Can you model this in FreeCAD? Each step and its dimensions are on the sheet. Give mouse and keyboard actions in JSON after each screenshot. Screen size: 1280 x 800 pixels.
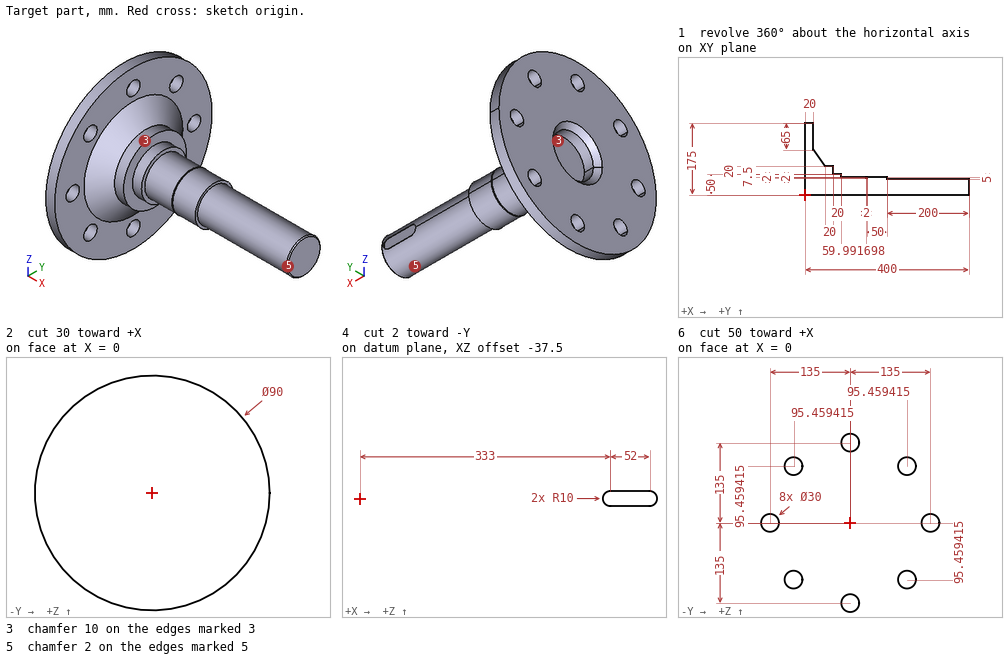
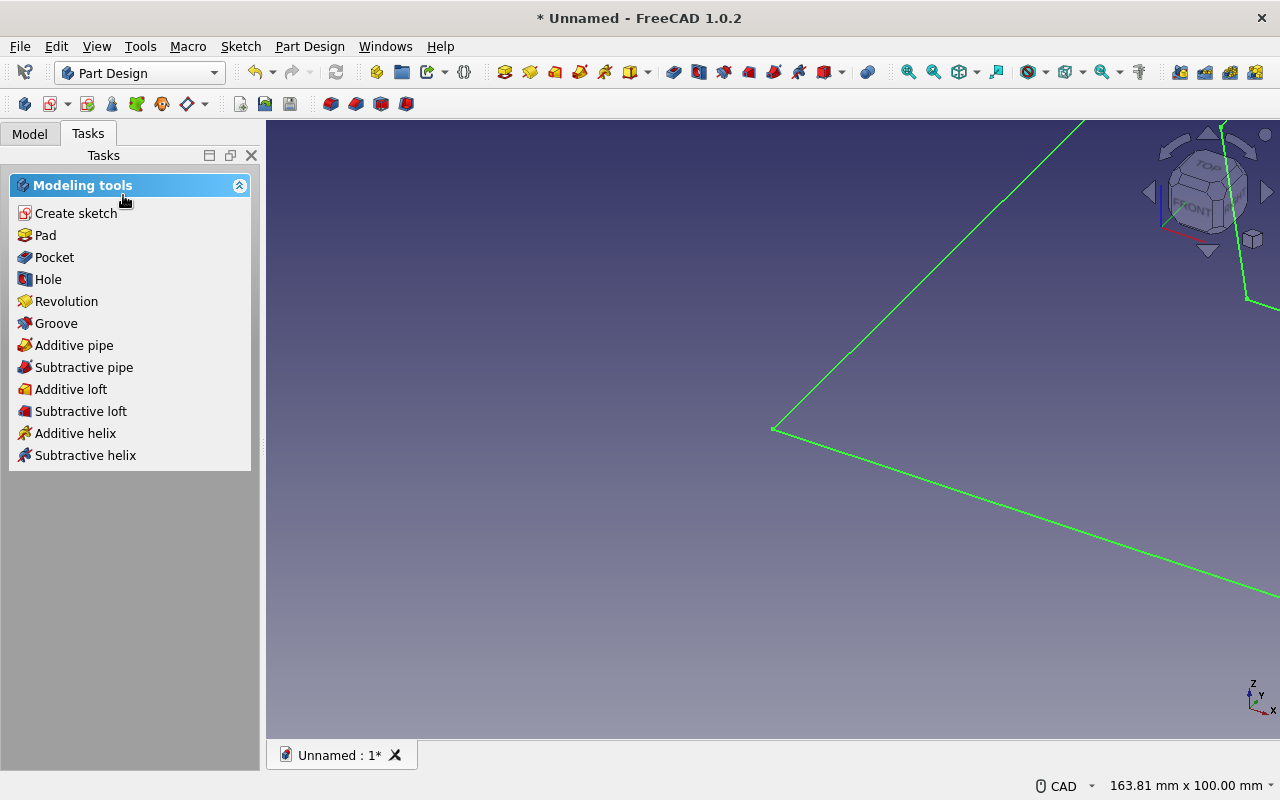
{"action": "left_click", "coordinate": [530, 72]}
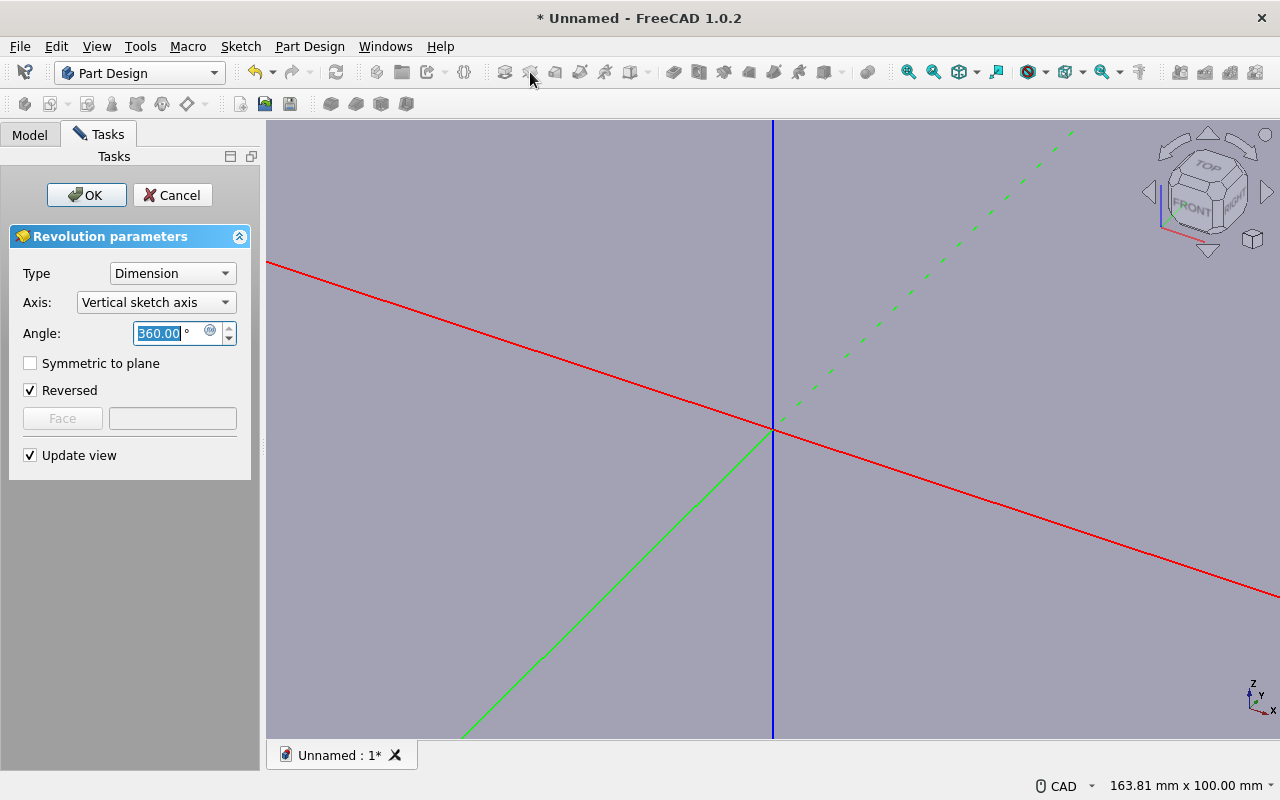
{"action": "left_click", "coordinate": [157, 302]}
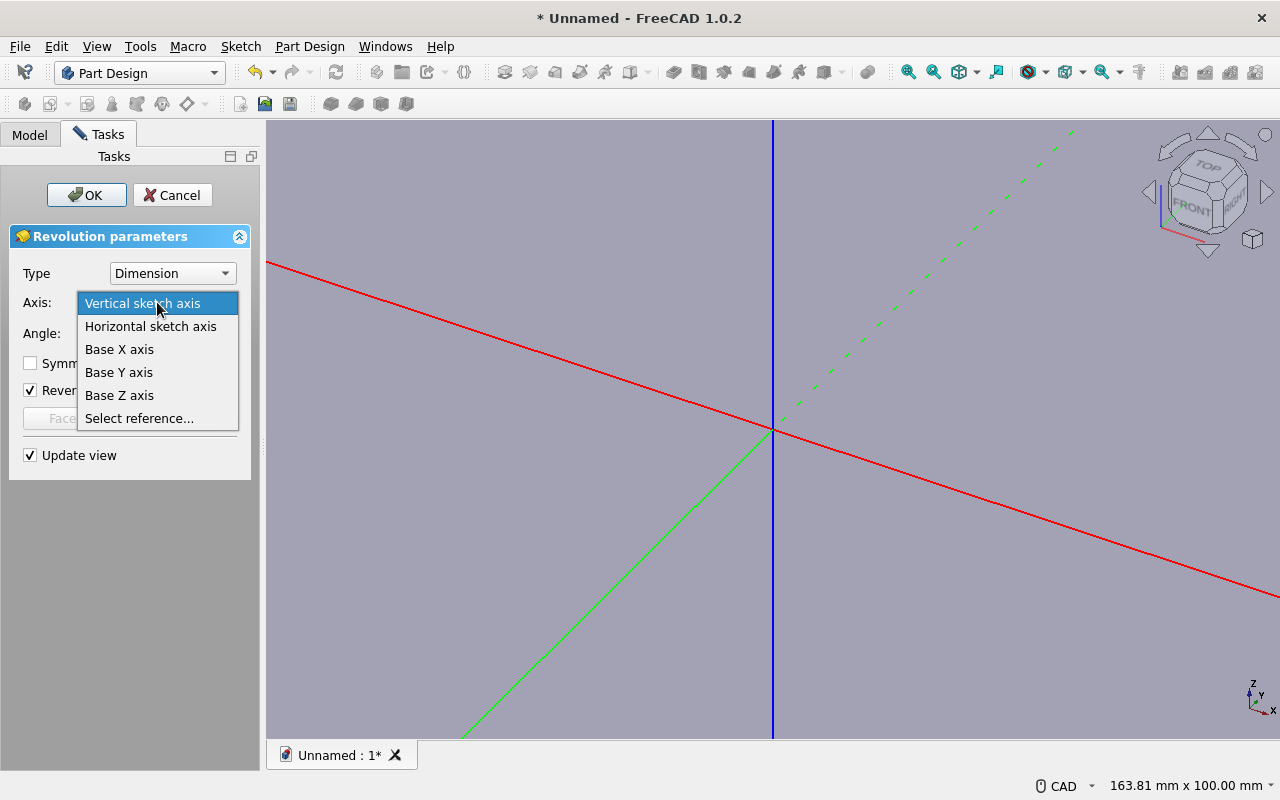
{"action": "left_click", "coordinate": [156, 326]}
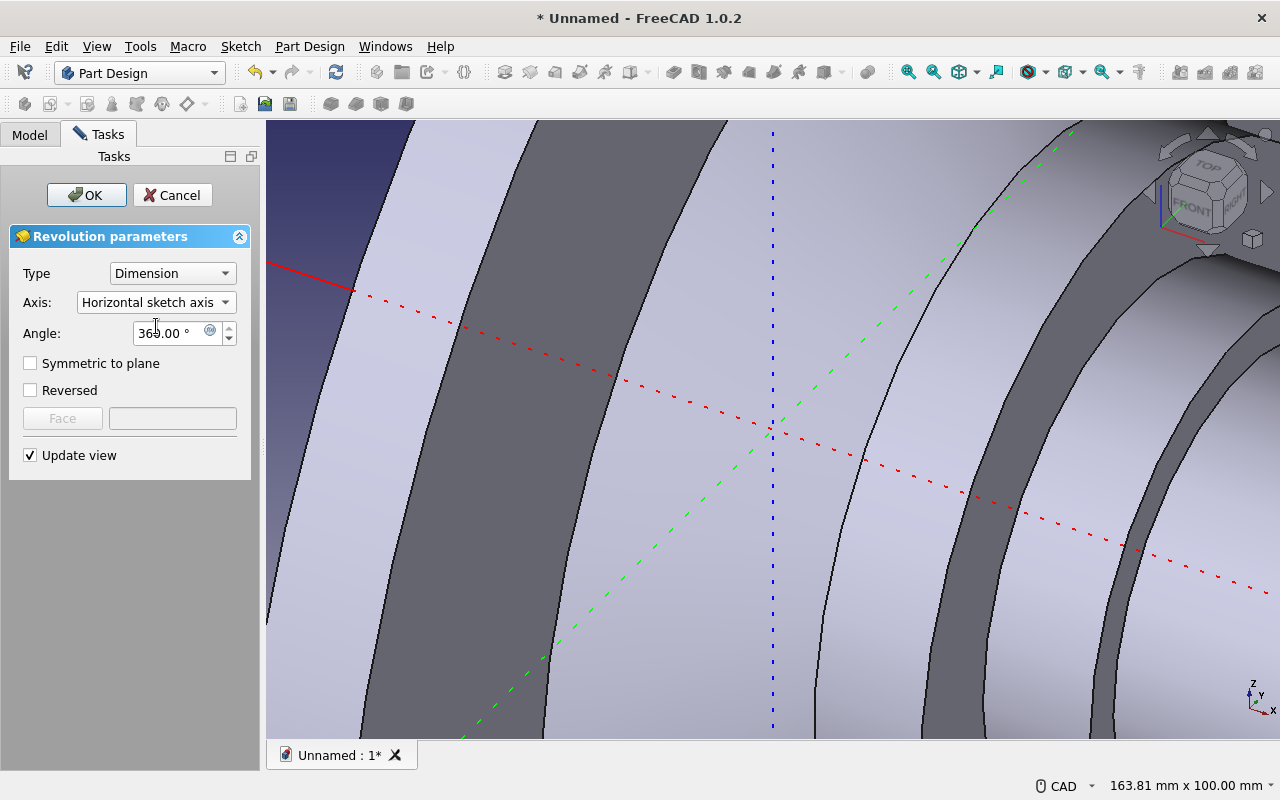
{"action": "left_click", "coordinate": [87, 195]}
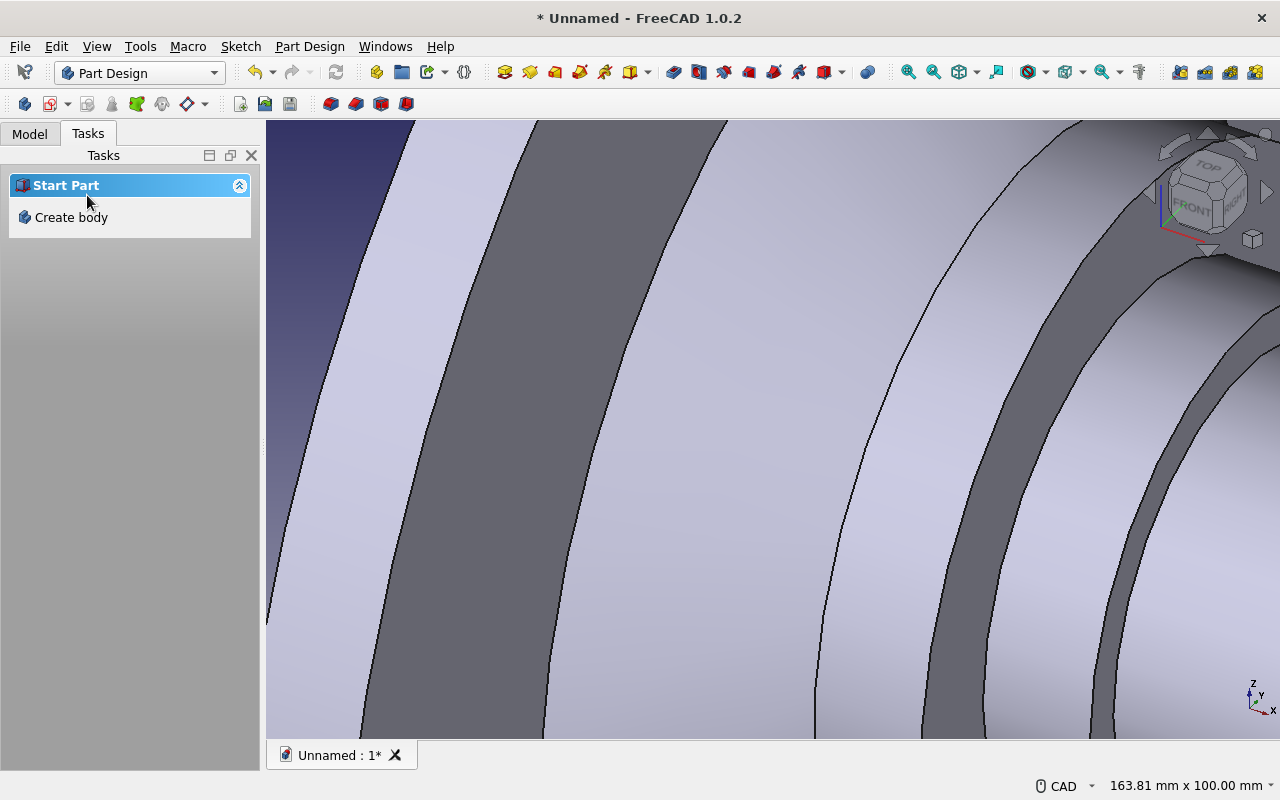
{"action": "left_click", "coordinate": [909, 72]}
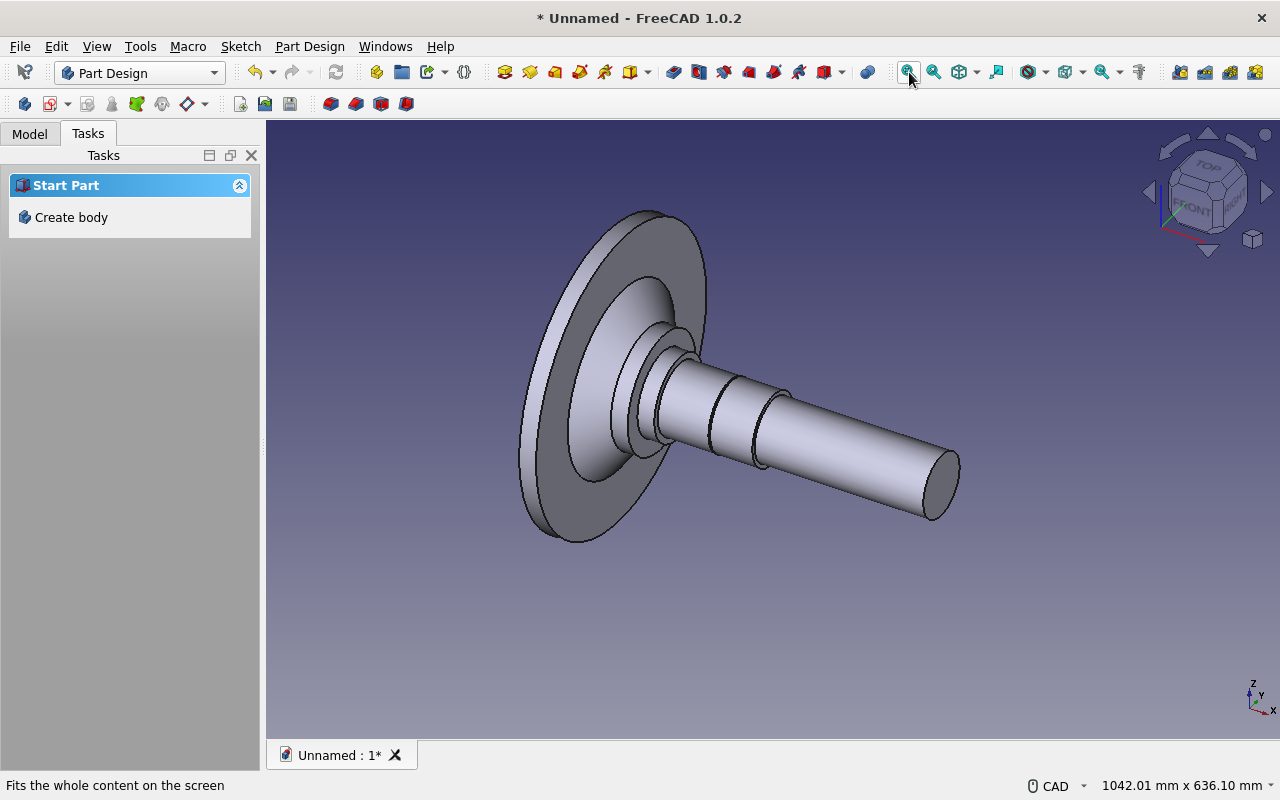
{"action": "key", "text": "6"}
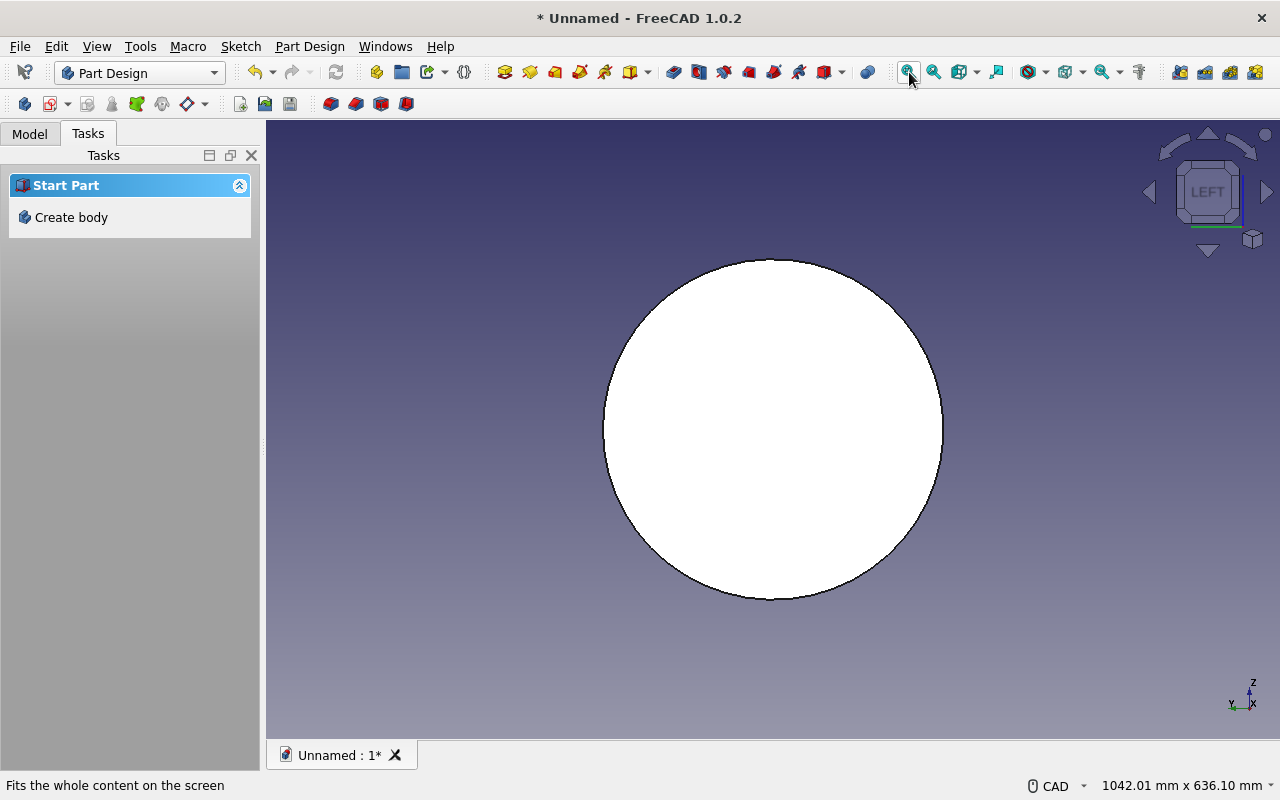
{"action": "left_click", "coordinate": [773, 428]}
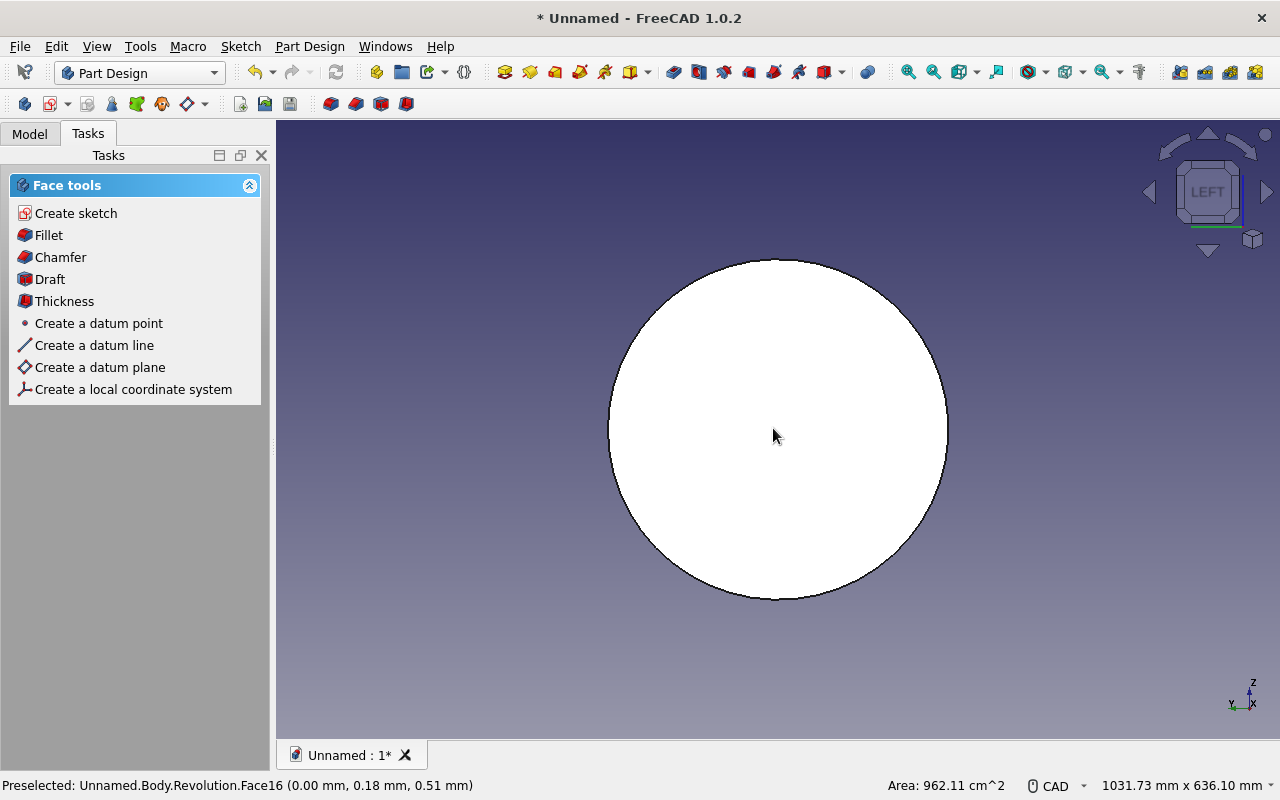
{"action": "left_click", "coordinate": [50, 104]}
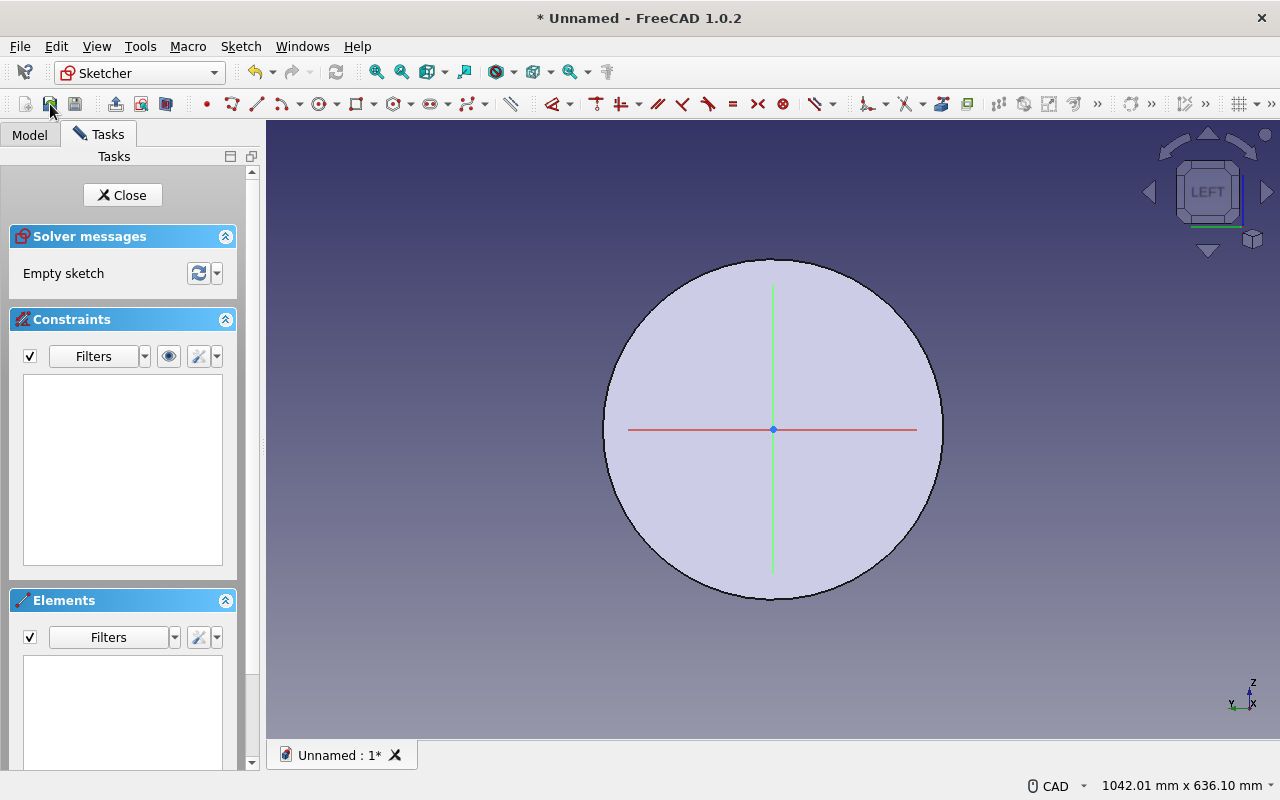
{"action": "scroll", "coordinate": [791, 430], "scroll_direction": "up", "scroll_amount": 8}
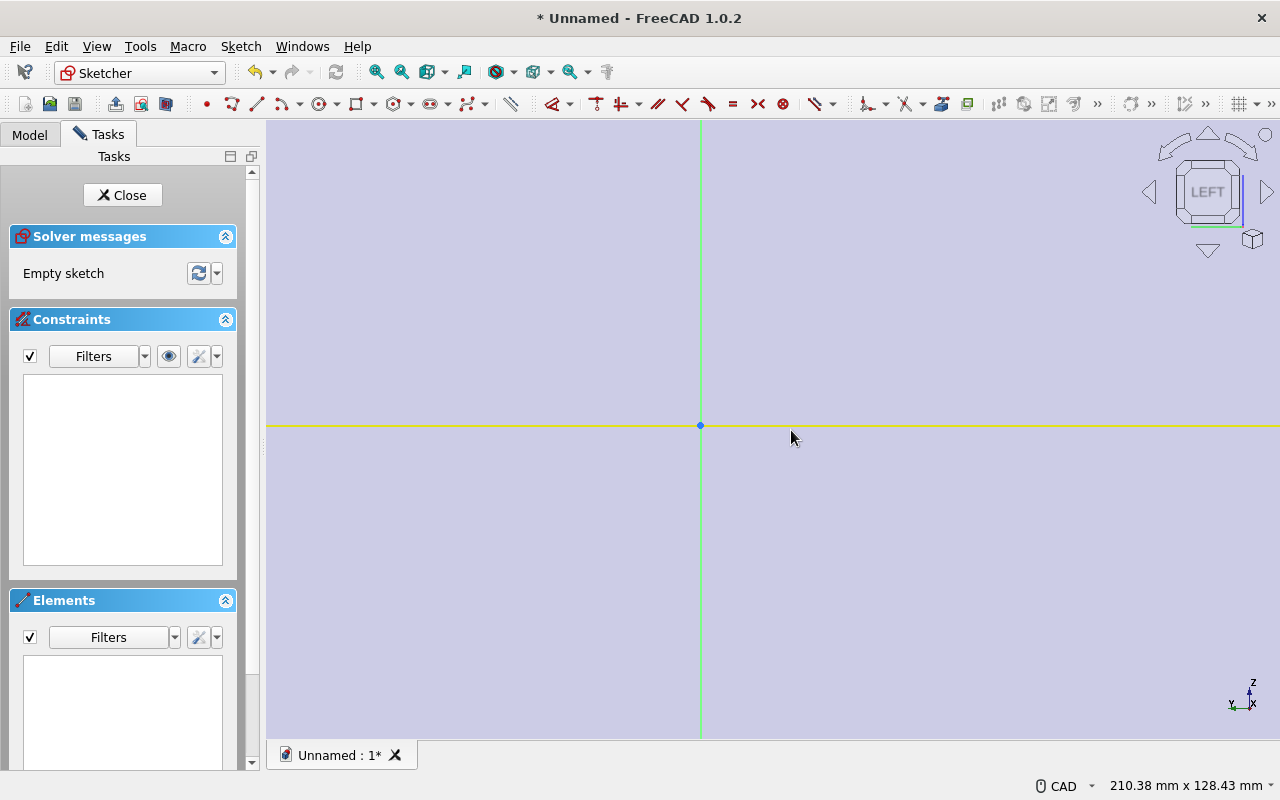
{"action": "left_click", "coordinate": [318, 104]}